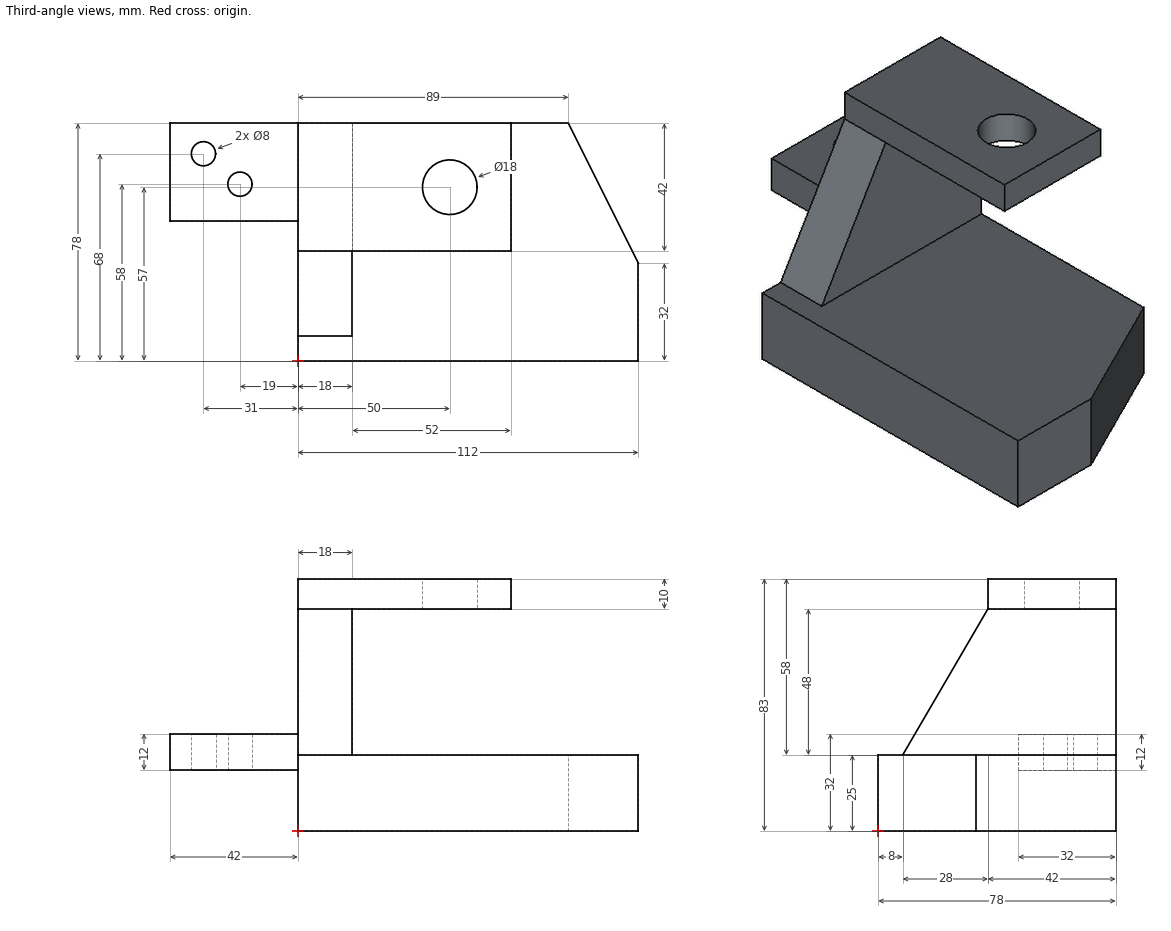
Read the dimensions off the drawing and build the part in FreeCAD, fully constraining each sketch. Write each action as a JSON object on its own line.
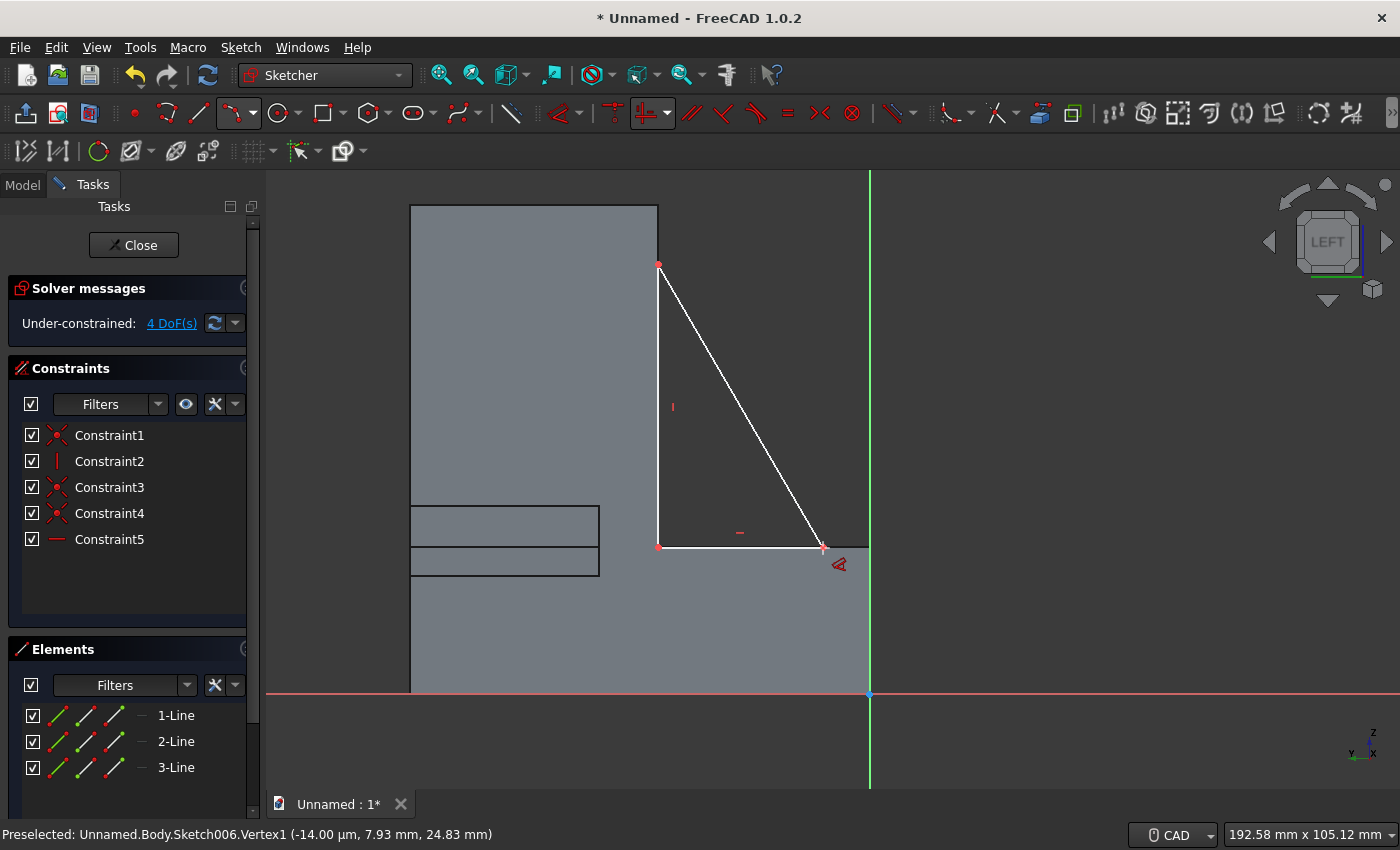
{"action": "left_click", "coordinate": [658, 350]}
{"action": "left_click", "coordinate": [624, 406]}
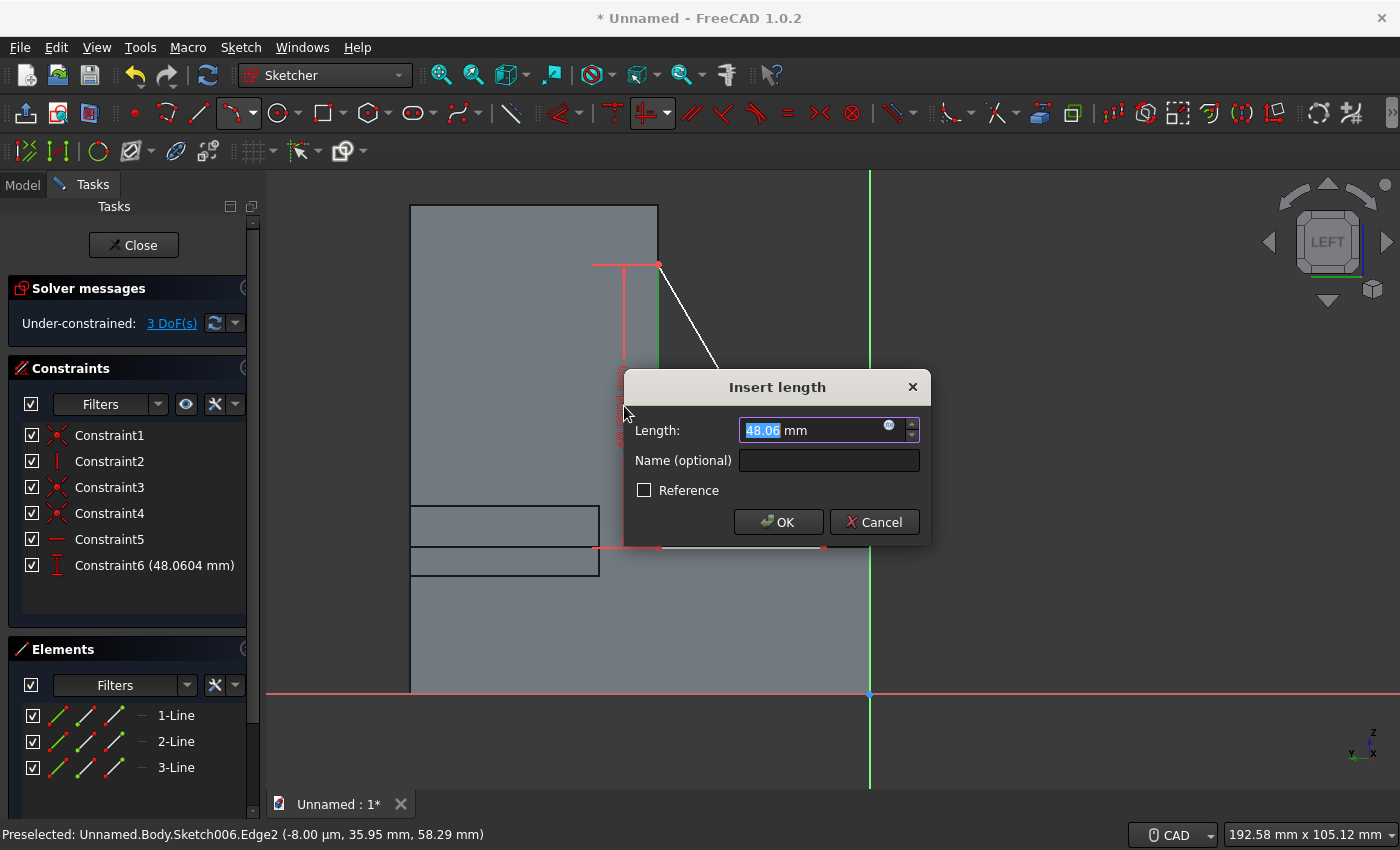
{"action": "type", "text": "48"}
{"action": "key", "text": "Return"}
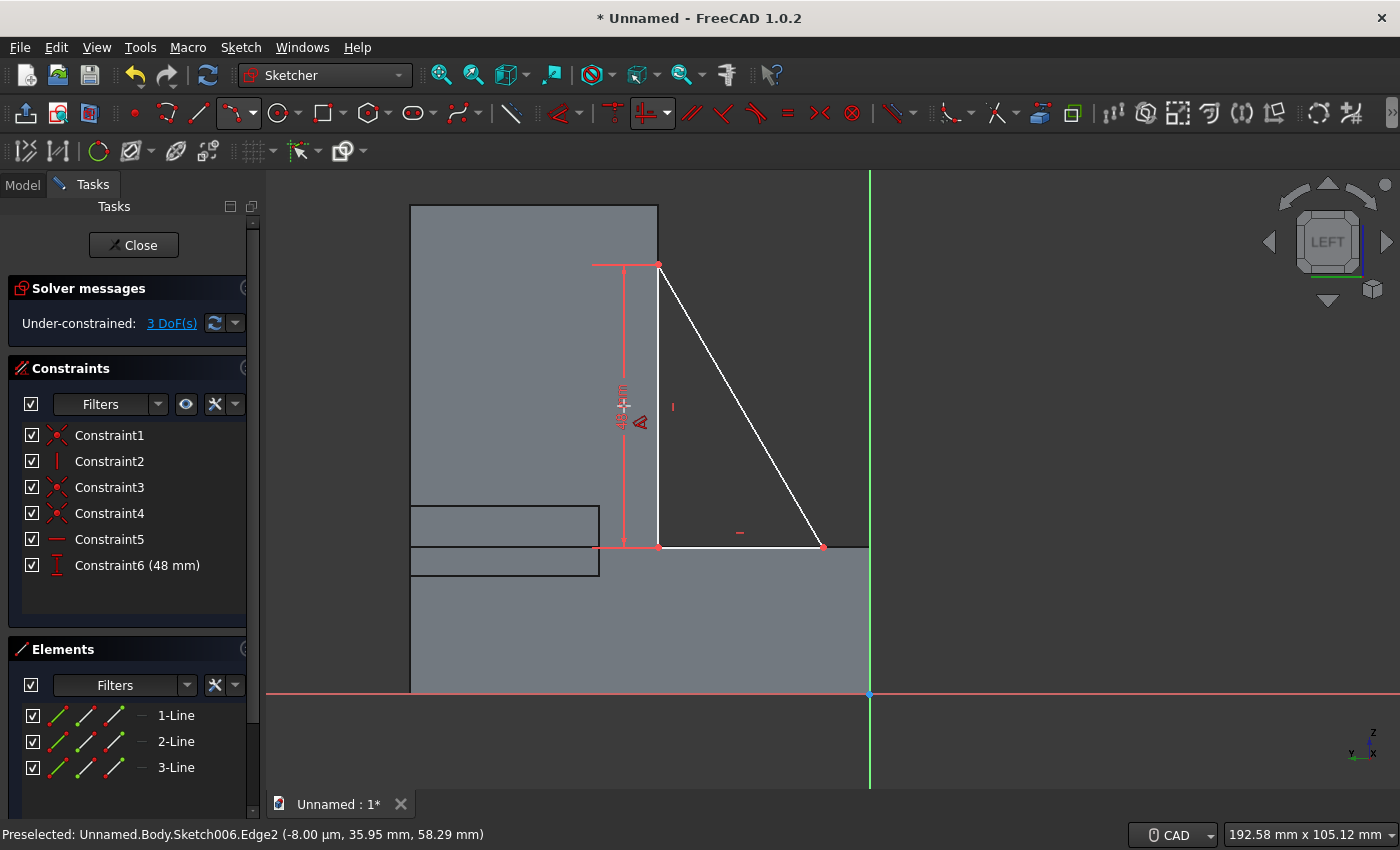
{"action": "left_click", "coordinate": [708, 548]}
{"action": "left_click", "coordinate": [741, 582]}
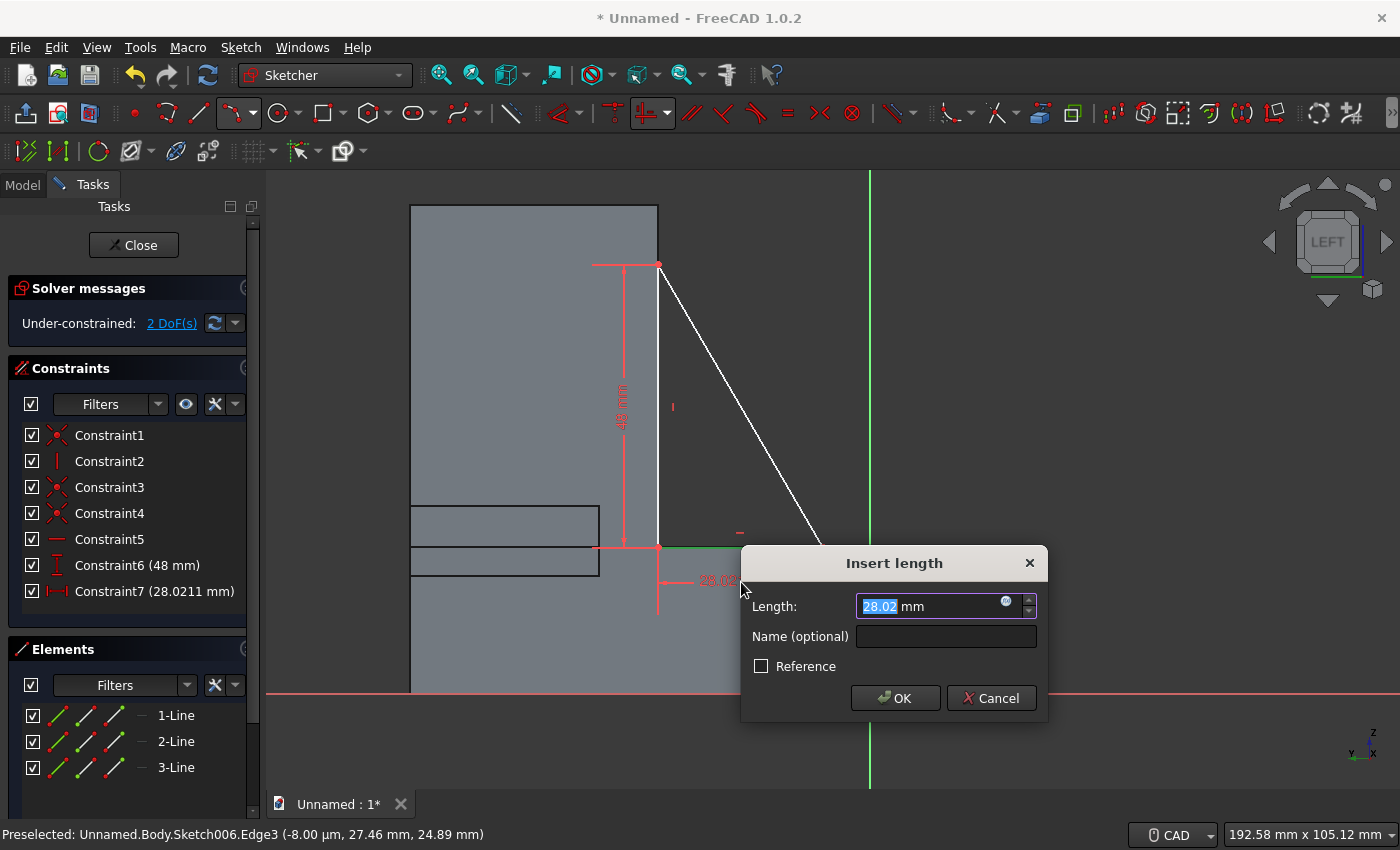
{"action": "type", "text": "28"}
{"action": "key", "text": "Return"}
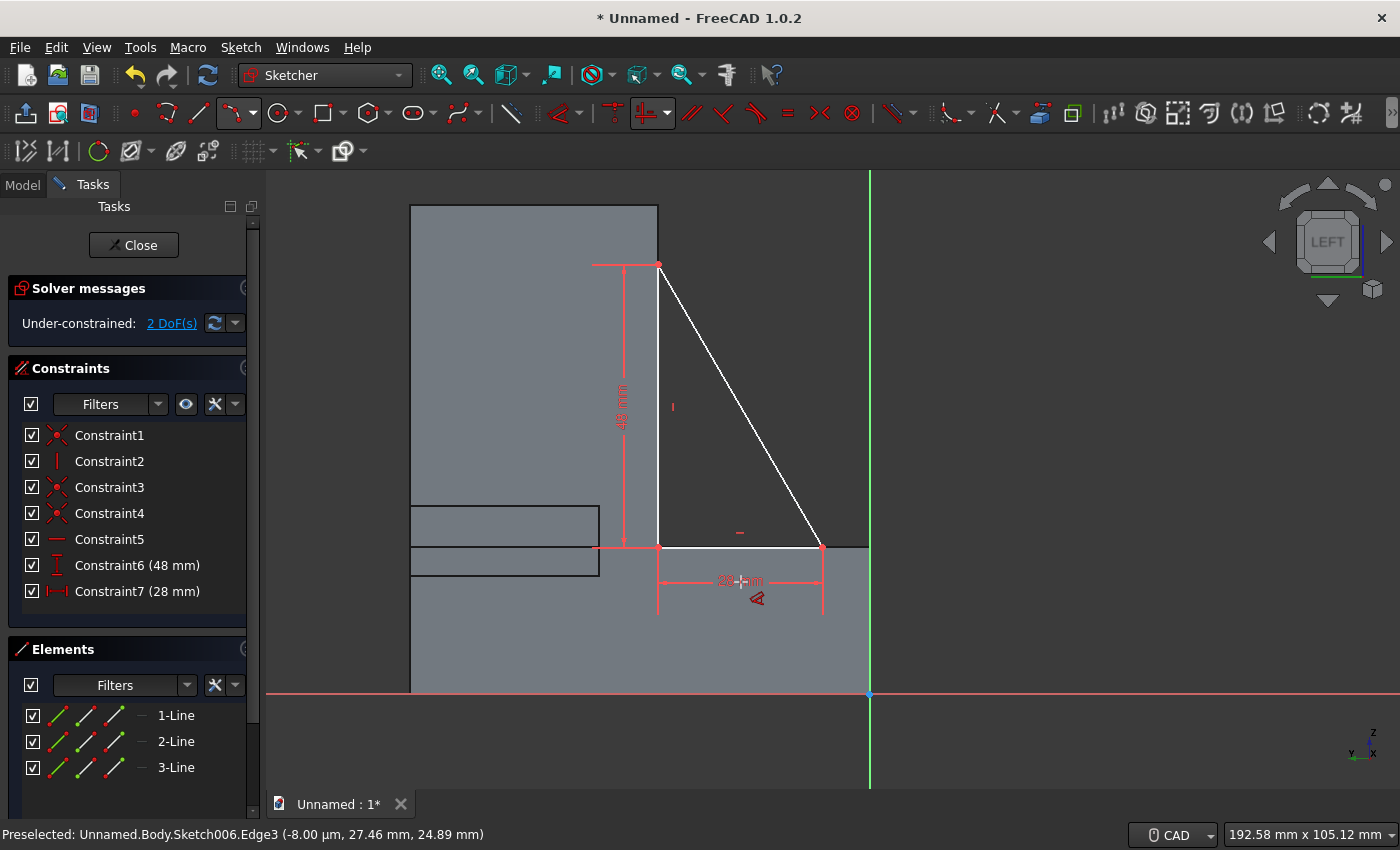
{"action": "left_click", "coordinate": [823, 548]}
{"action": "left_click", "coordinate": [846, 728]}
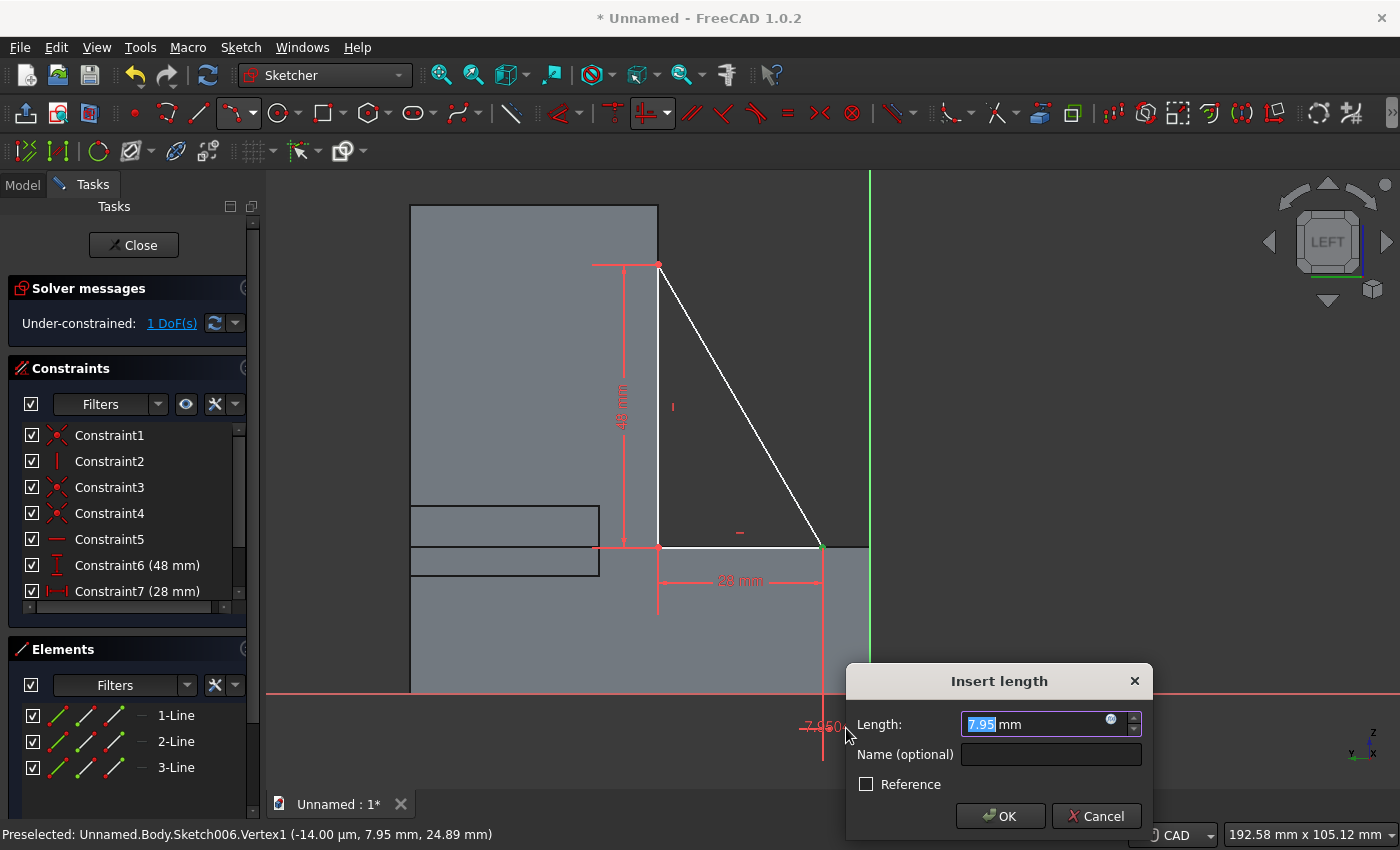
{"action": "type", "text": "8"}
{"action": "key", "text": "Return"}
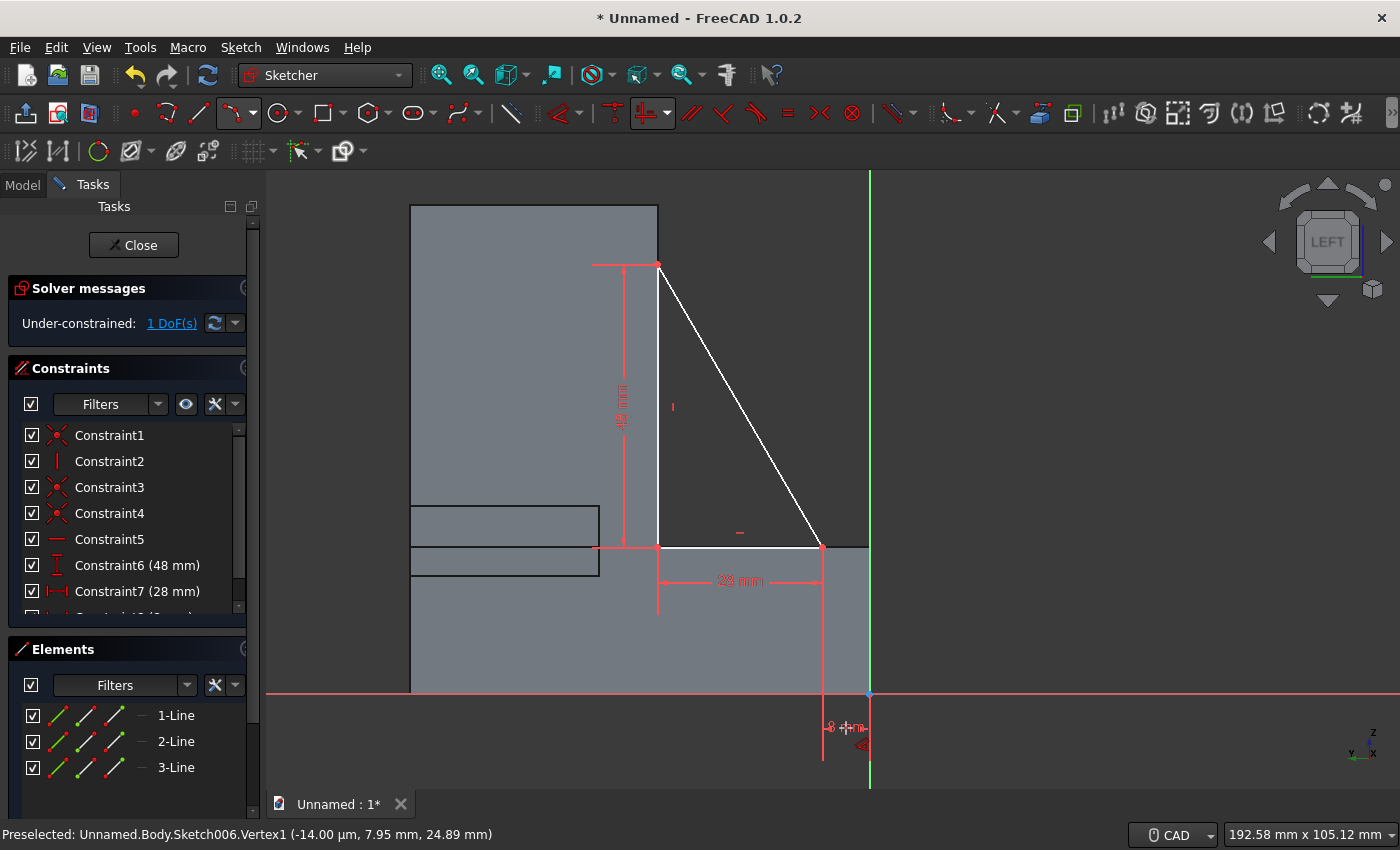
{"action": "left_click", "coordinate": [823, 548]}
{"action": "left_click", "coordinate": [904, 621]}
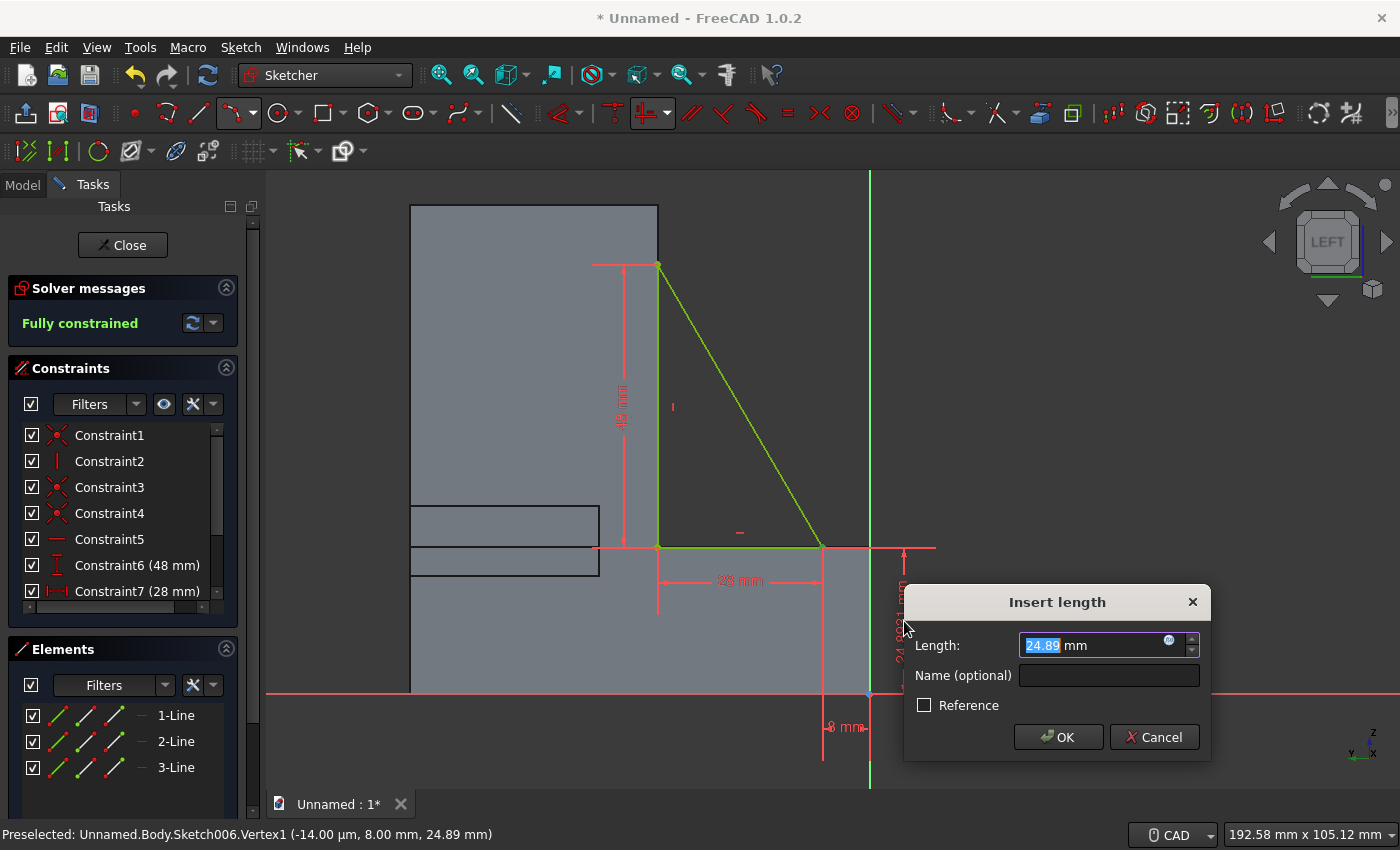
{"action": "type", "text": "25"}
{"action": "key", "text": "Return"}
{"action": "key", "text": "Escape"}